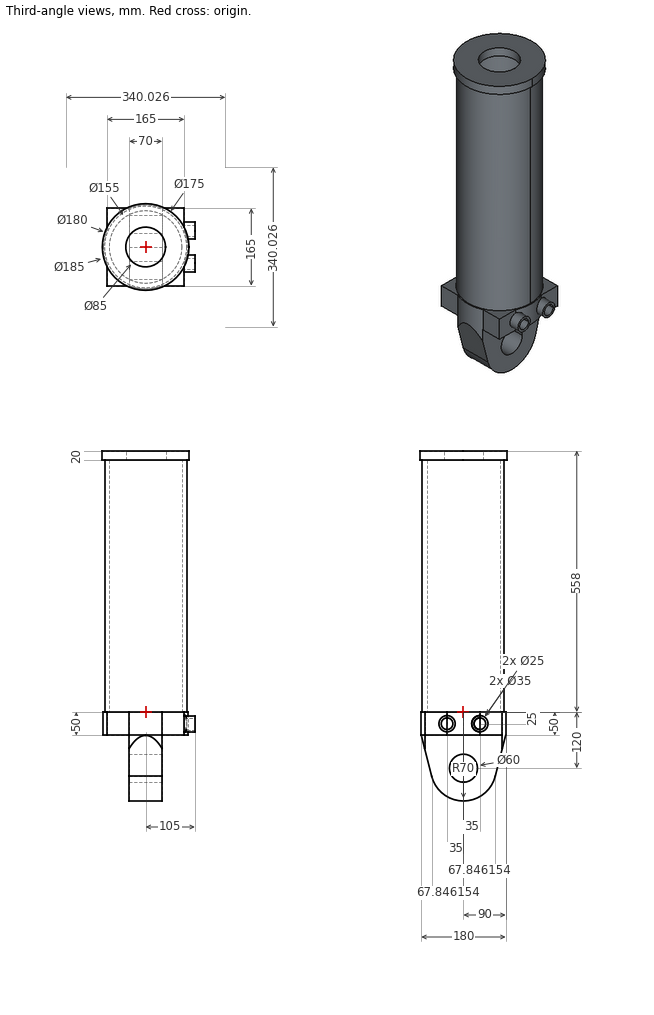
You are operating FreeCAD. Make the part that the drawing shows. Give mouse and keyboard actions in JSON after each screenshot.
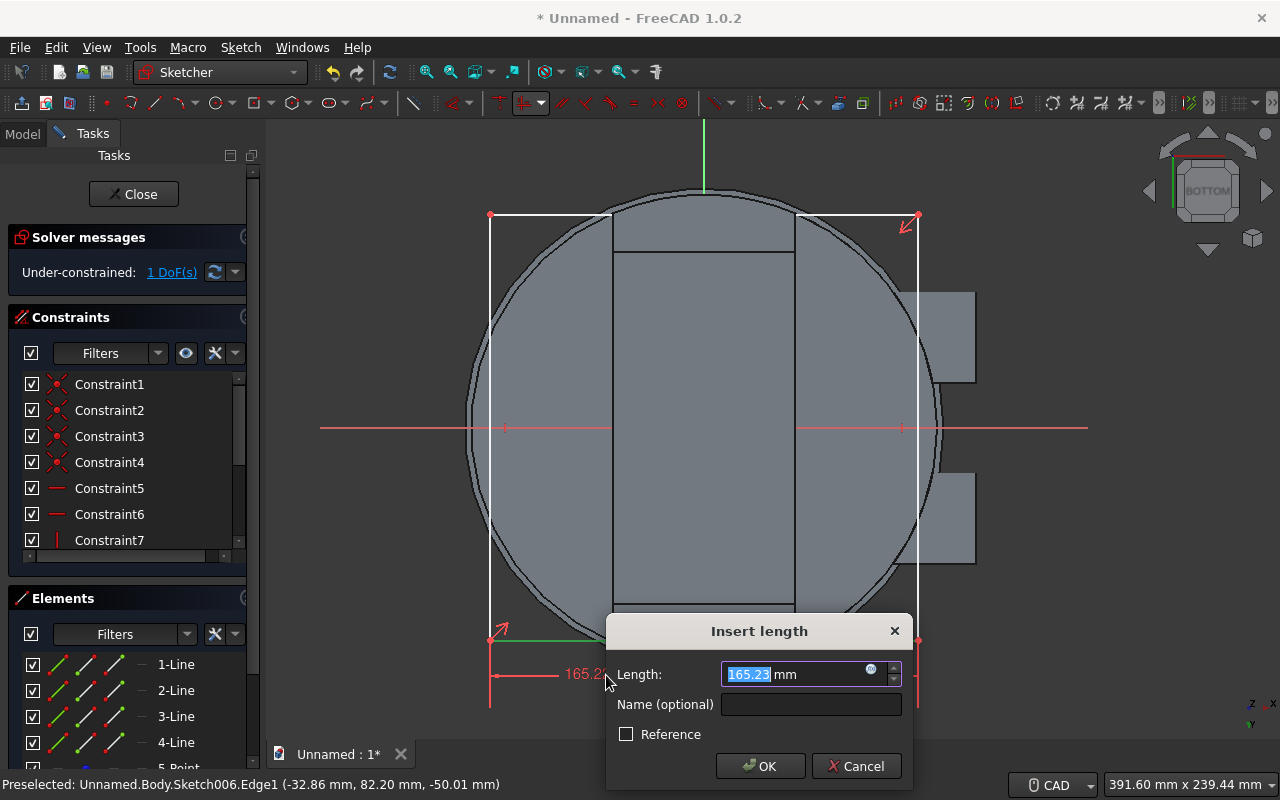
{"action": "type", "text": "165"}
{"action": "key", "text": "Return"}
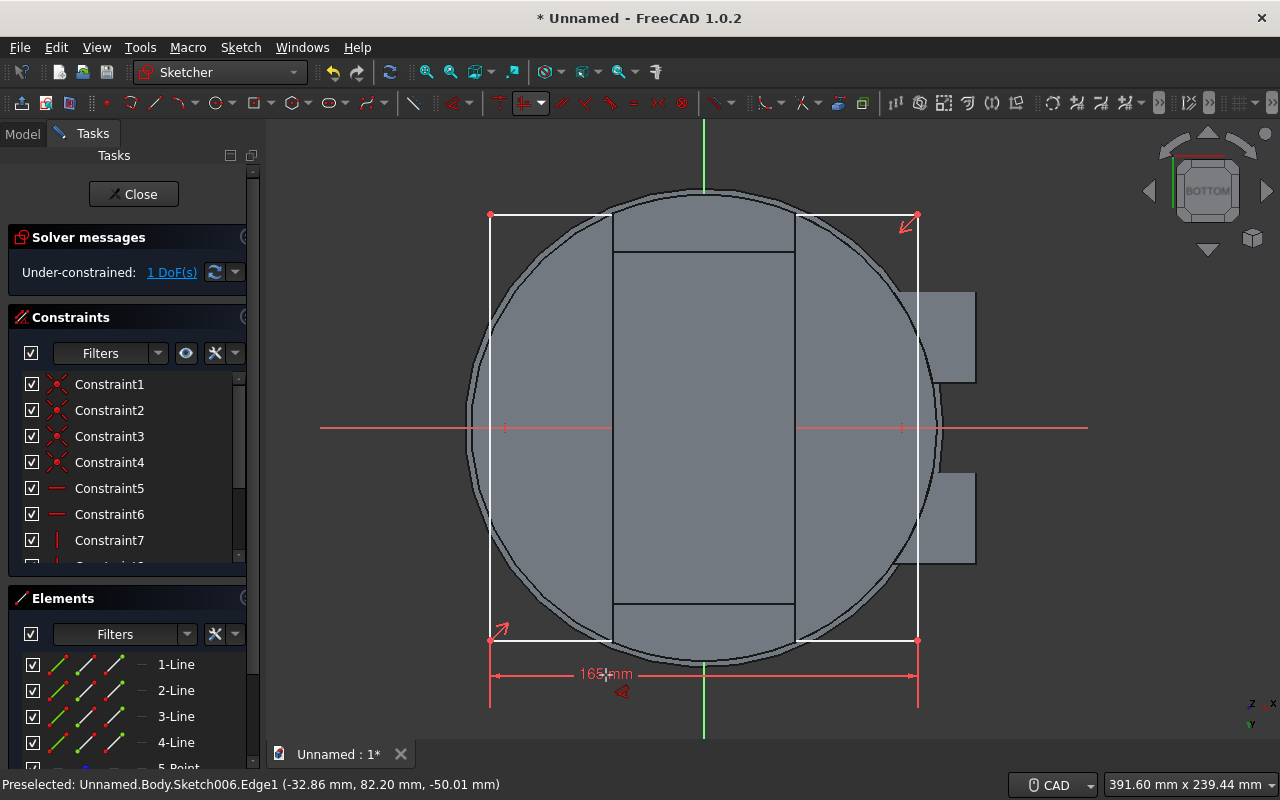
{"action": "left_click", "coordinate": [918, 513]}
{"action": "left_click", "coordinate": [952, 330]}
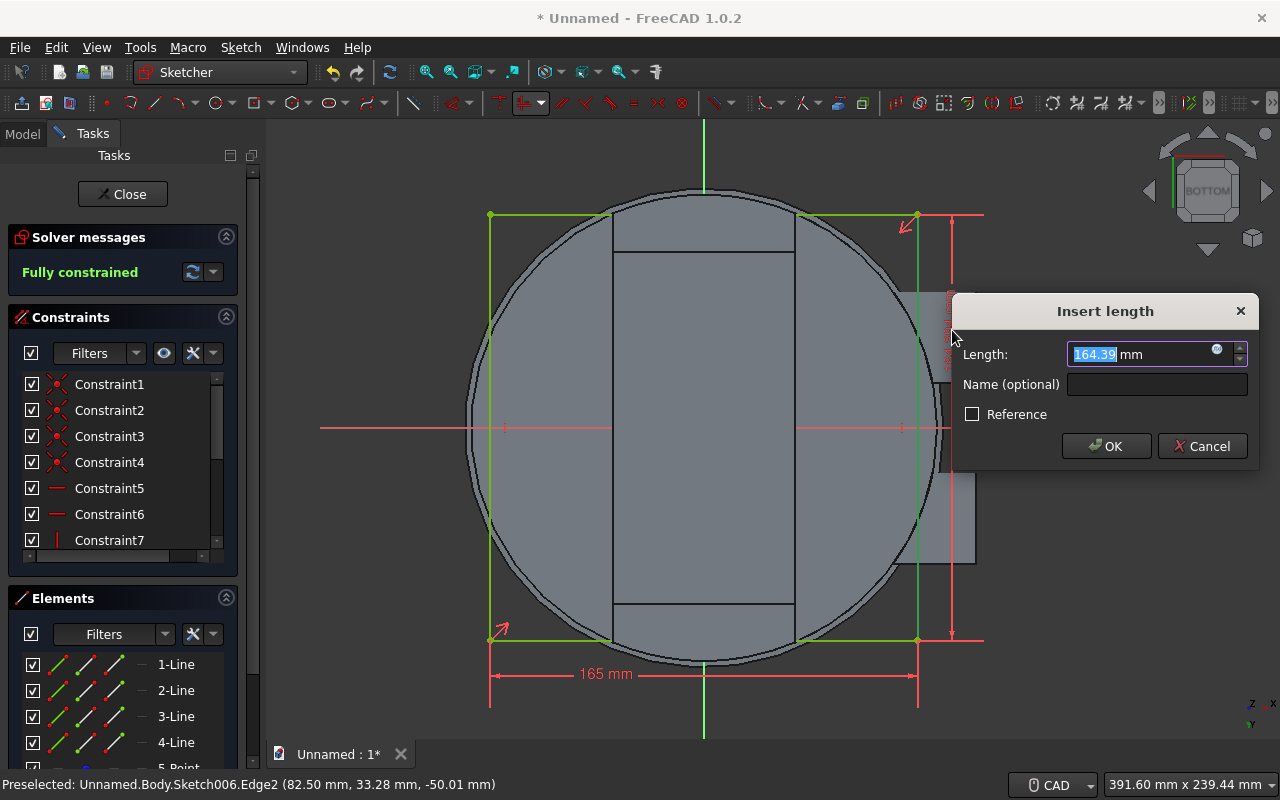
{"action": "type", "text": "165"}
{"action": "key", "text": "Return"}
{"action": "key", "text": "Escape"}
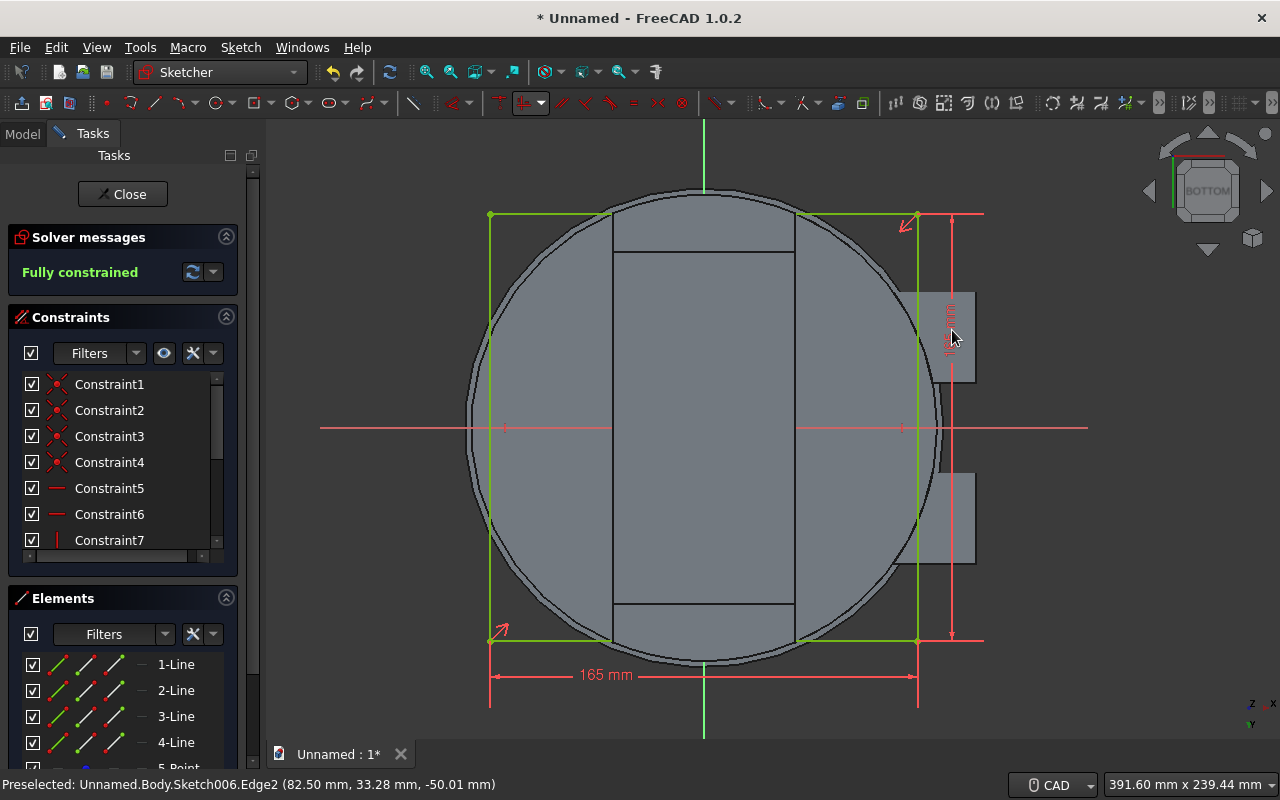
{"action": "left_click", "coordinate": [123, 194]}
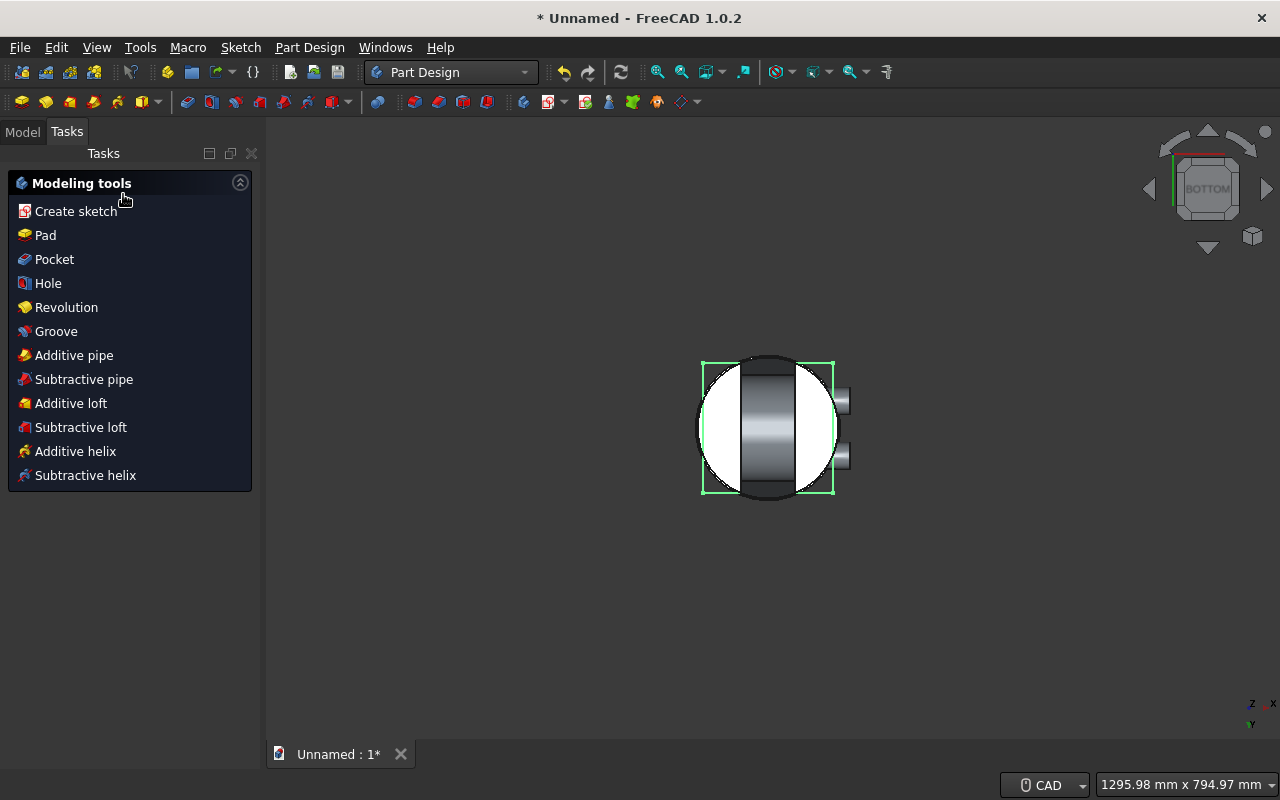
{"action": "left_click", "coordinate": [22, 102]}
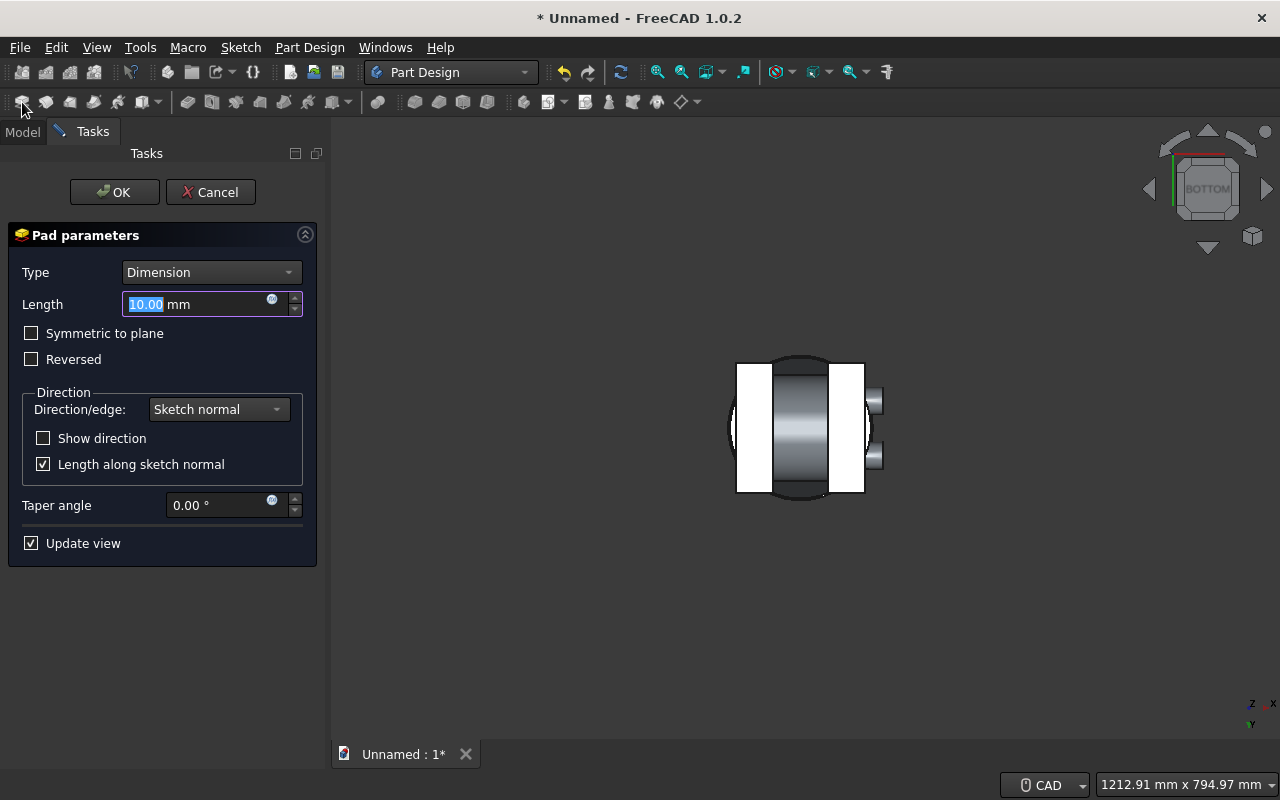
{"action": "type", "text": "50"}
{"action": "key", "text": "Tab"}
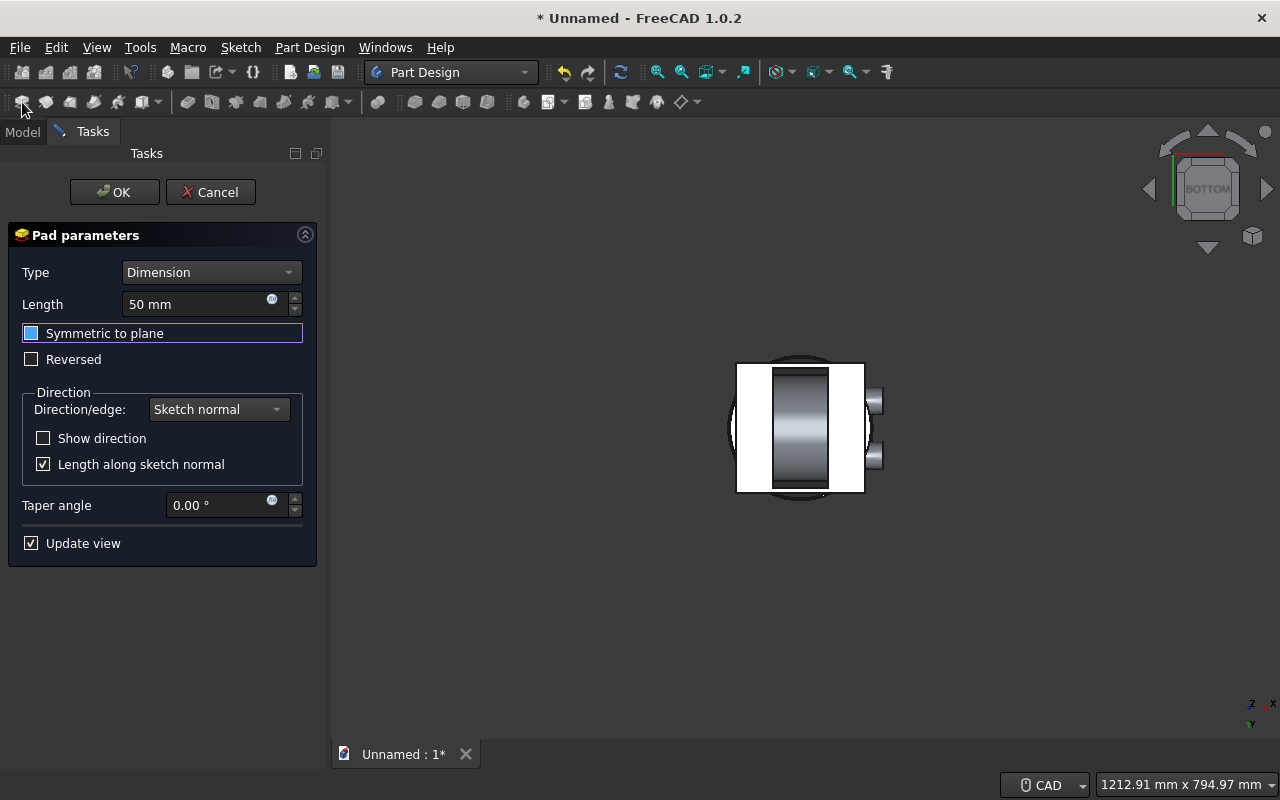
{"action": "left_click", "coordinate": [30, 359]}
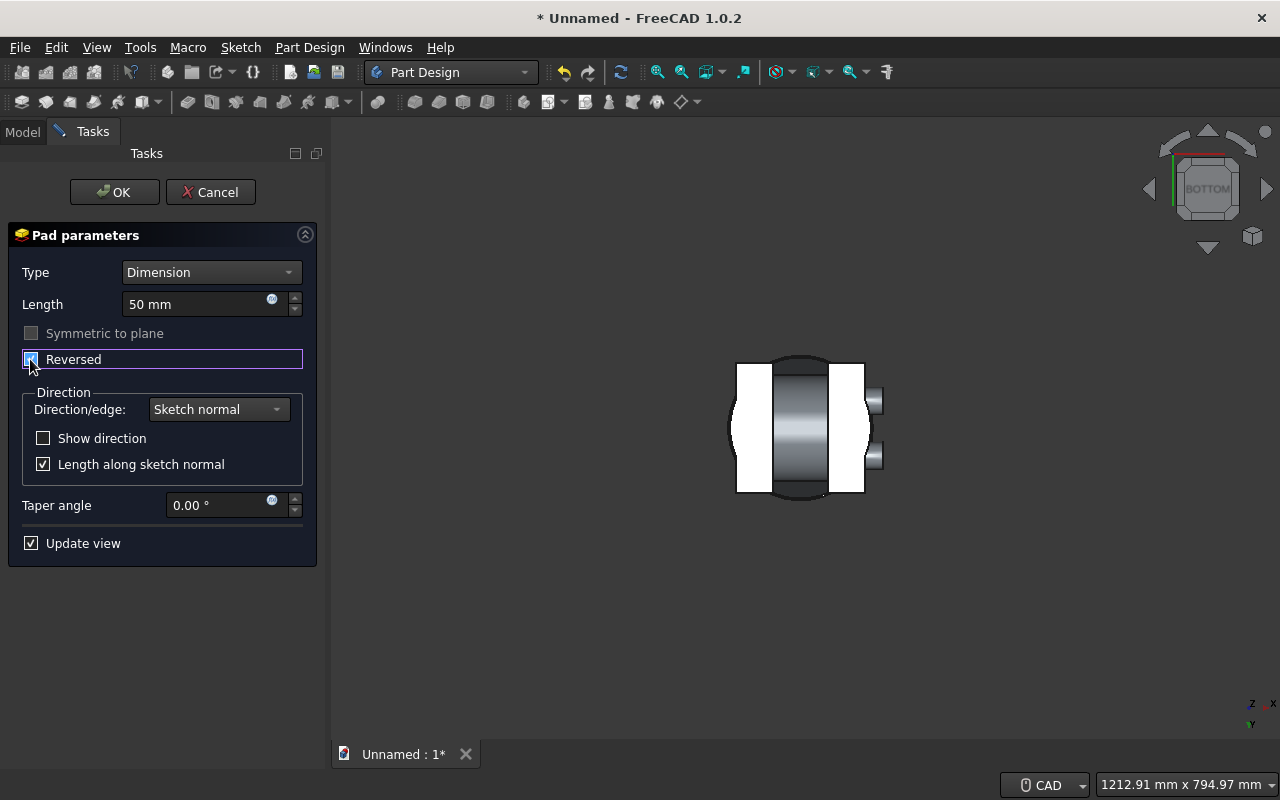
{"action": "left_click", "coordinate": [115, 192]}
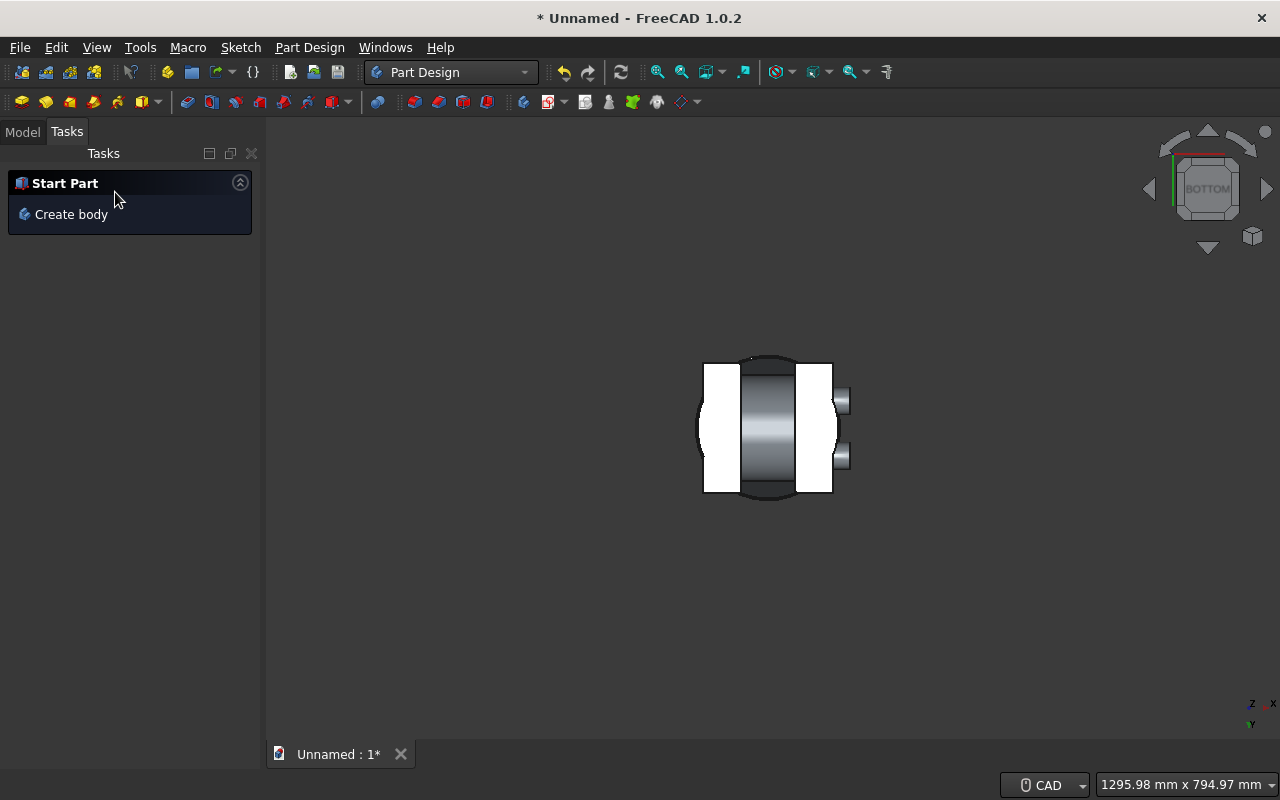
{"action": "key", "text": "0"}